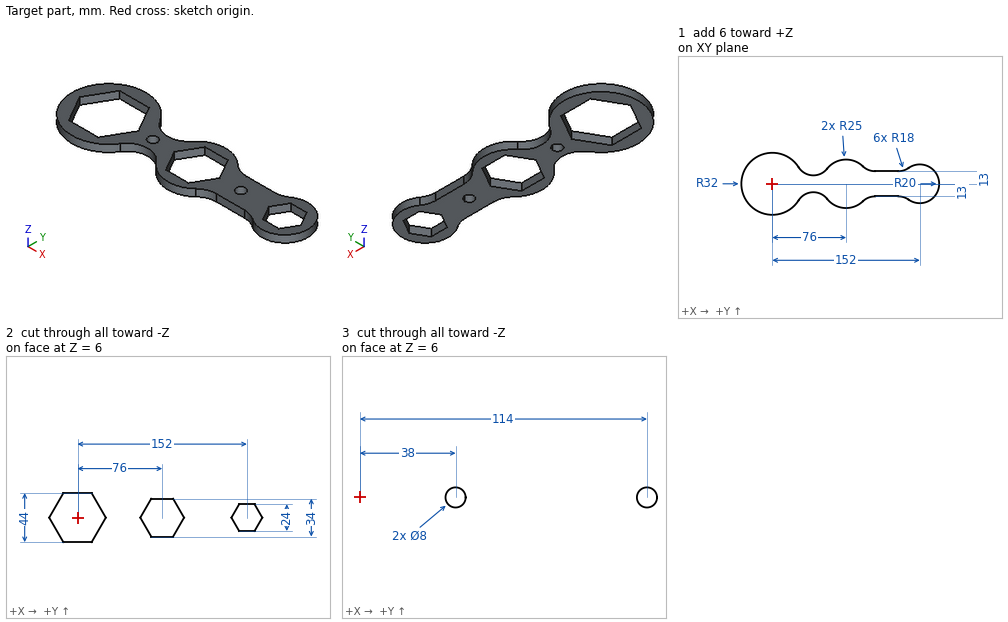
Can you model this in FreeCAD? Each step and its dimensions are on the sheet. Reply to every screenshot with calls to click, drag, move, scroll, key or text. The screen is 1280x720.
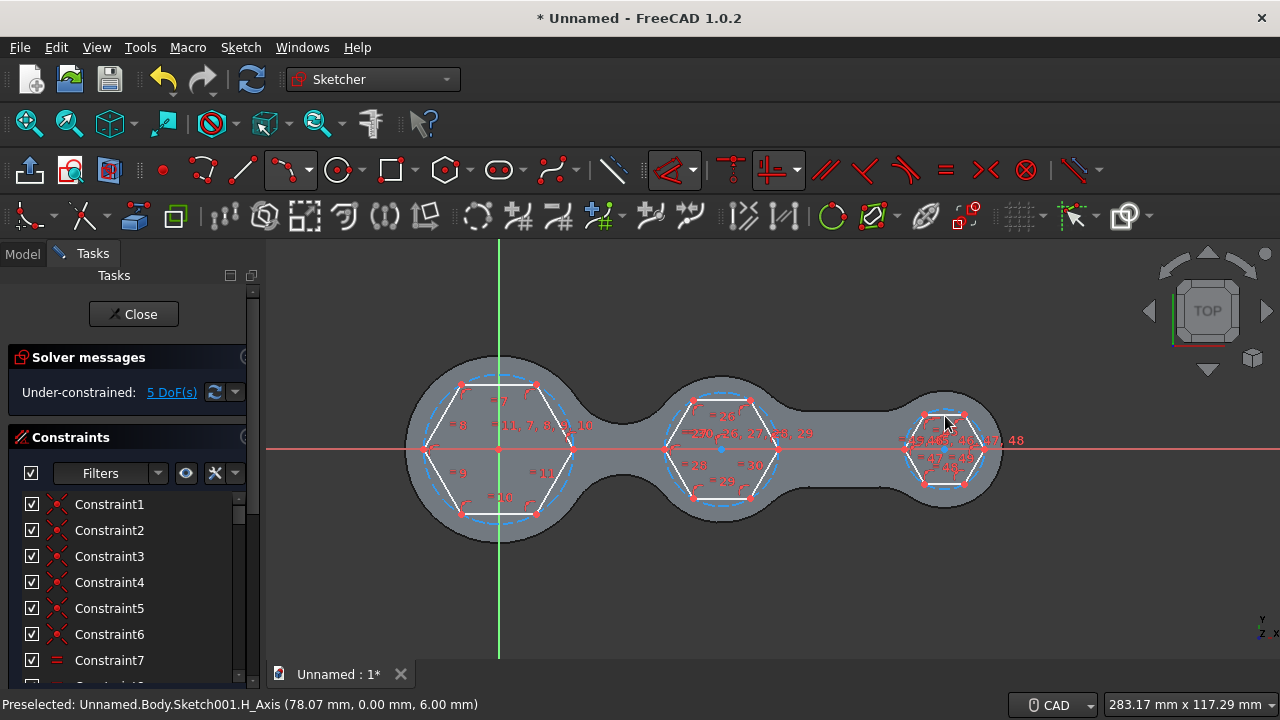
click(461, 514)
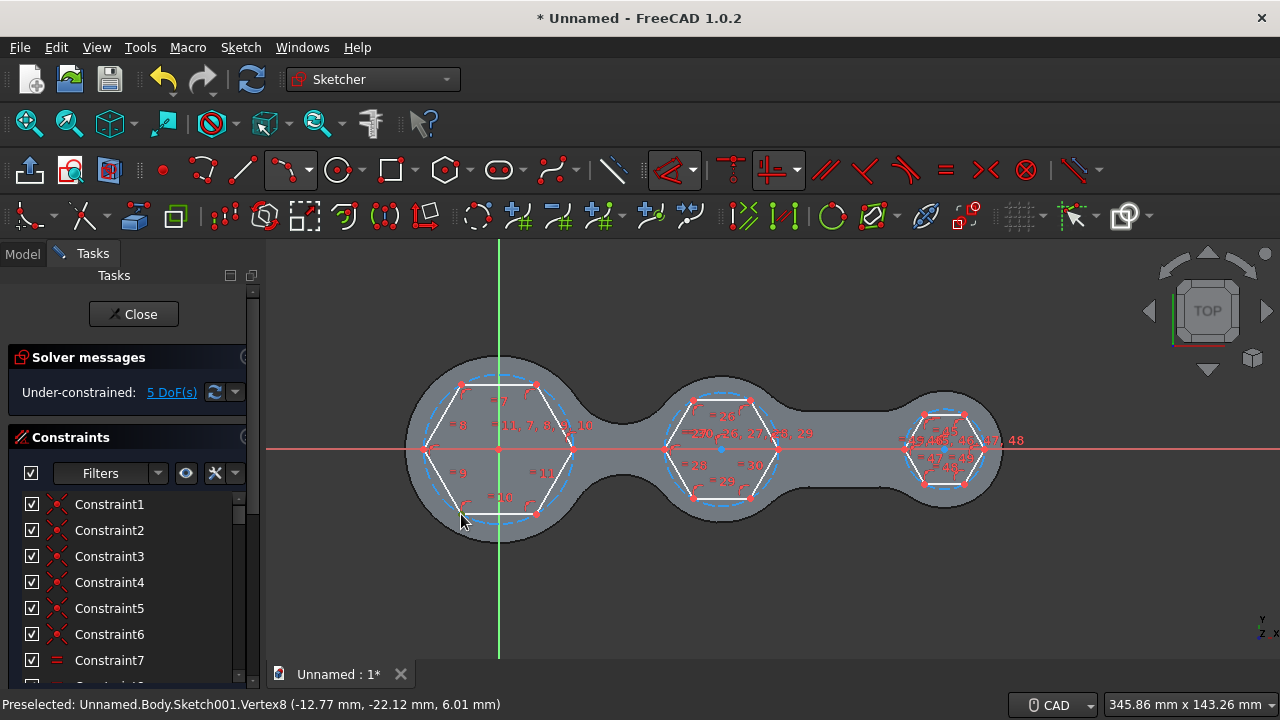
click(536, 385)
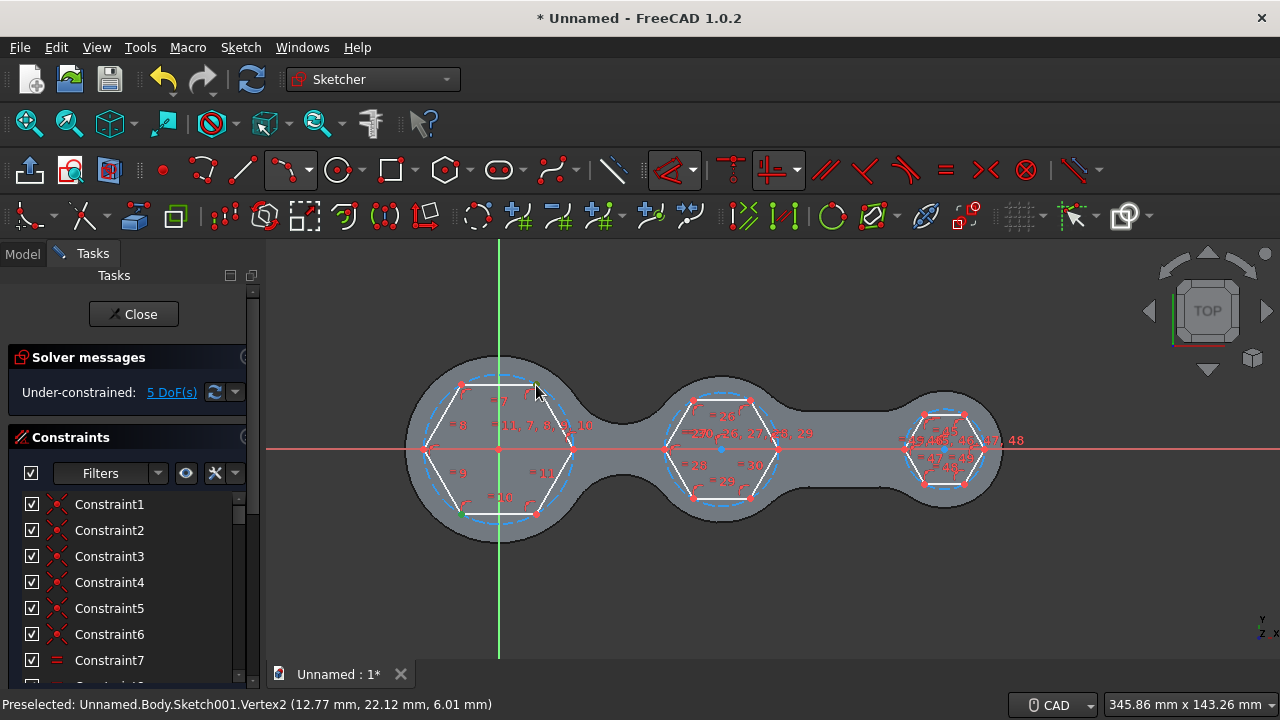
click(696, 170)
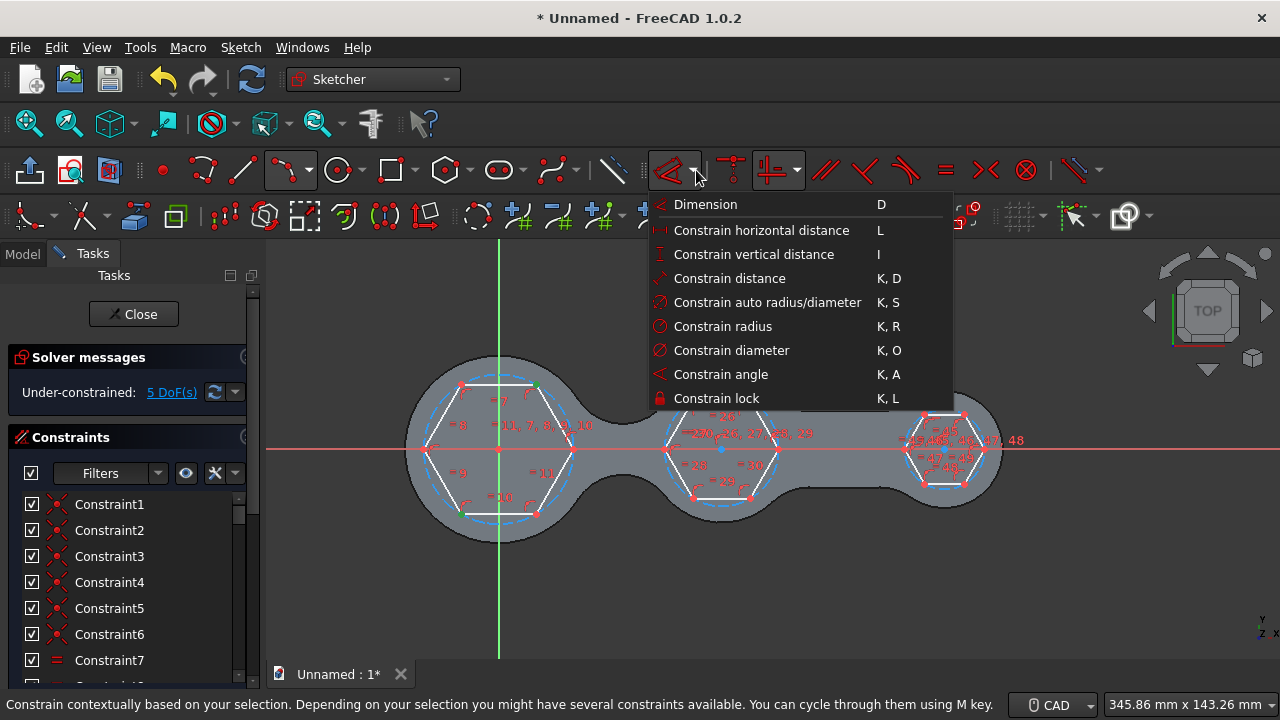
click(801, 254)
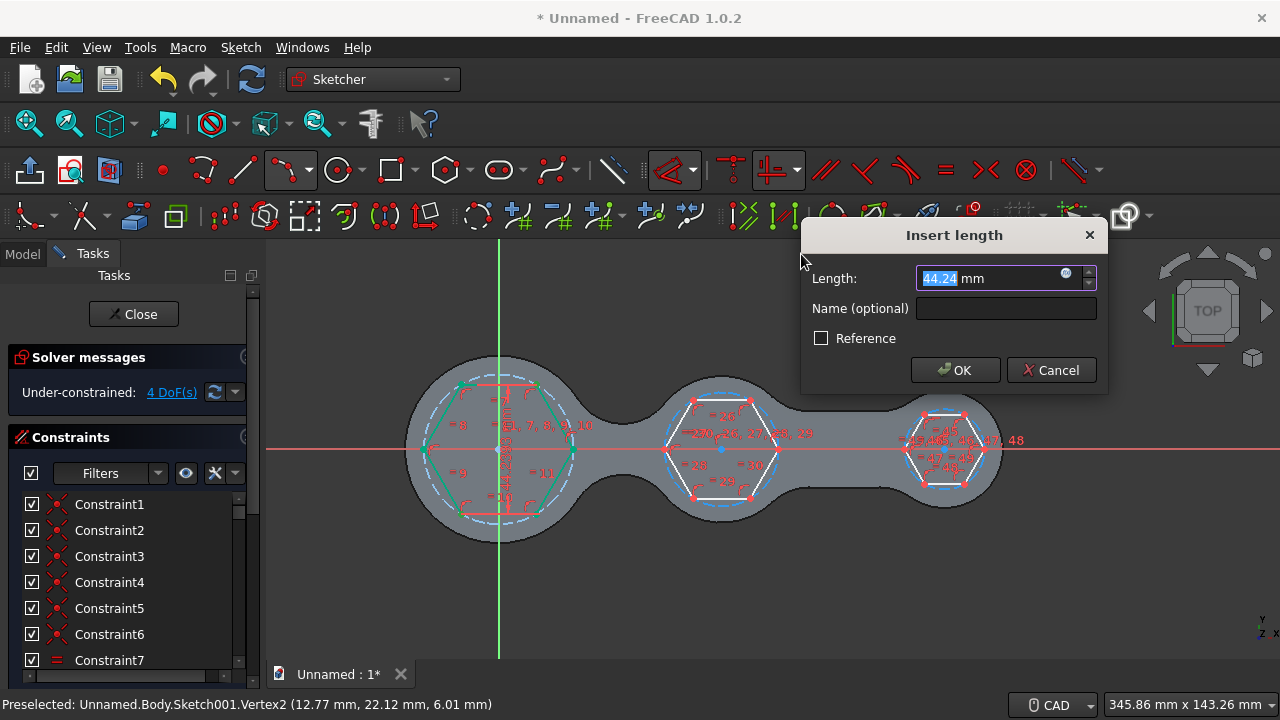
text(44)
key(Return)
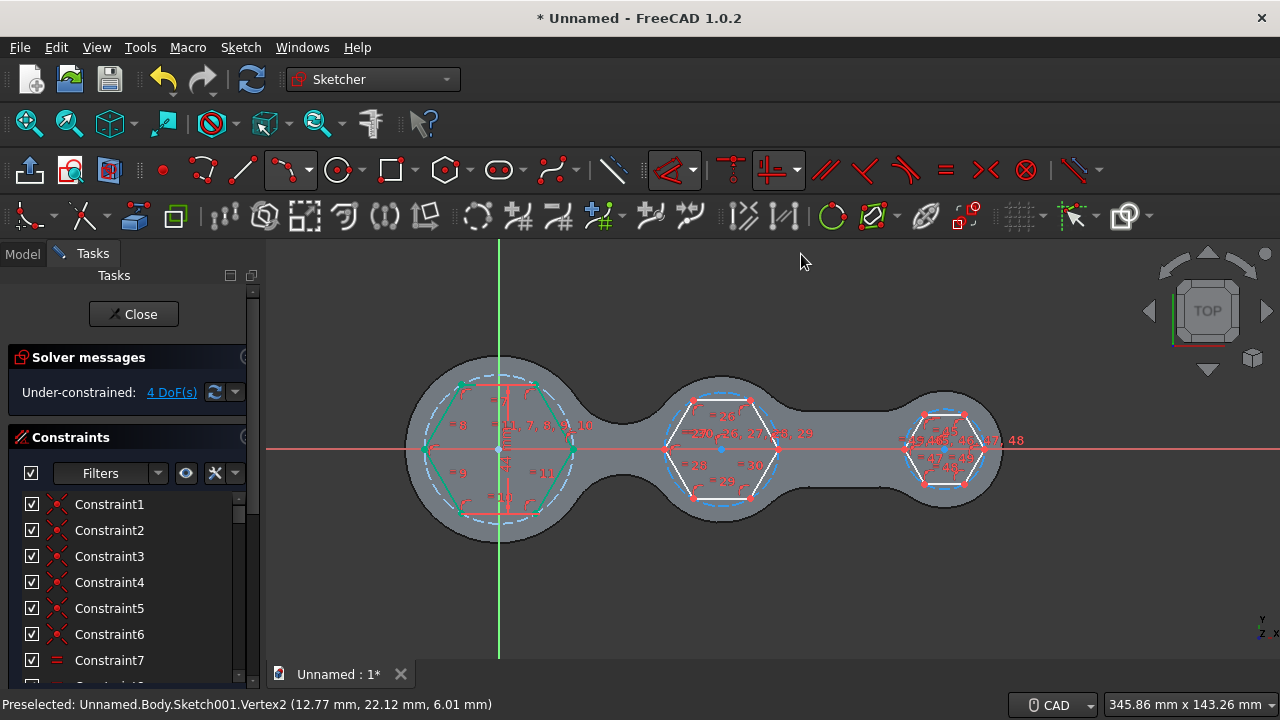
click(693, 499)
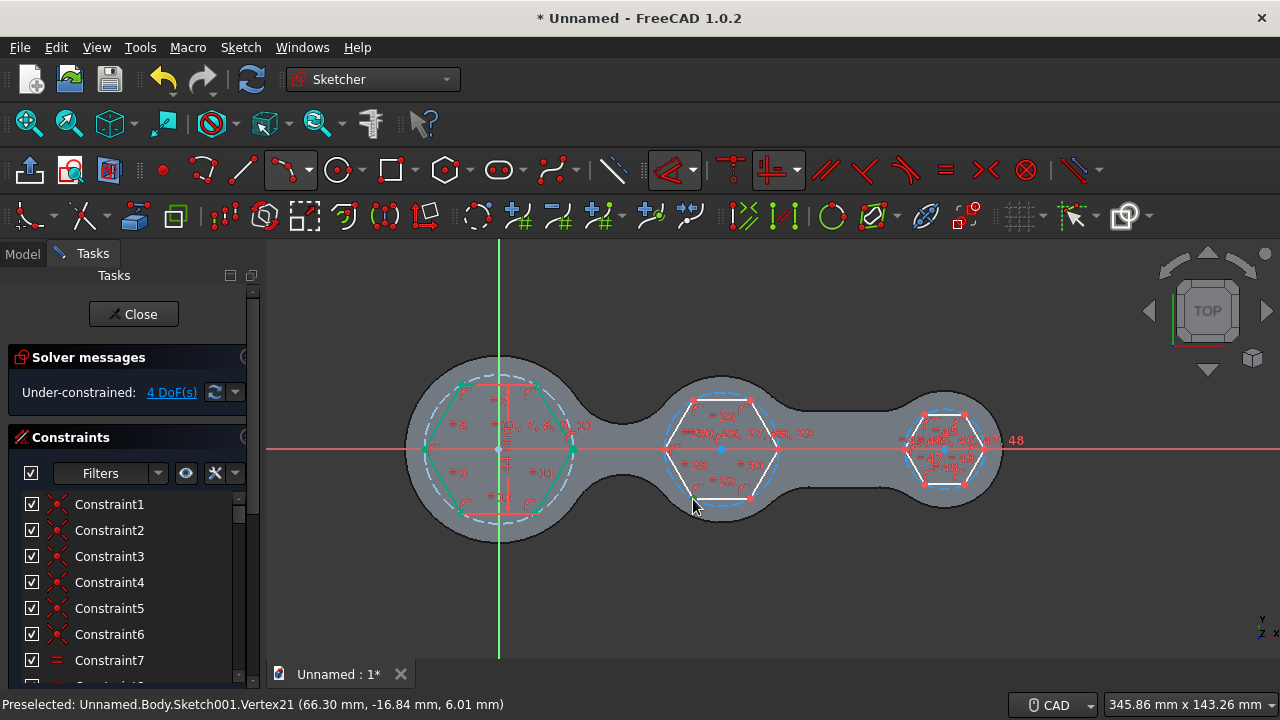
click(750, 400)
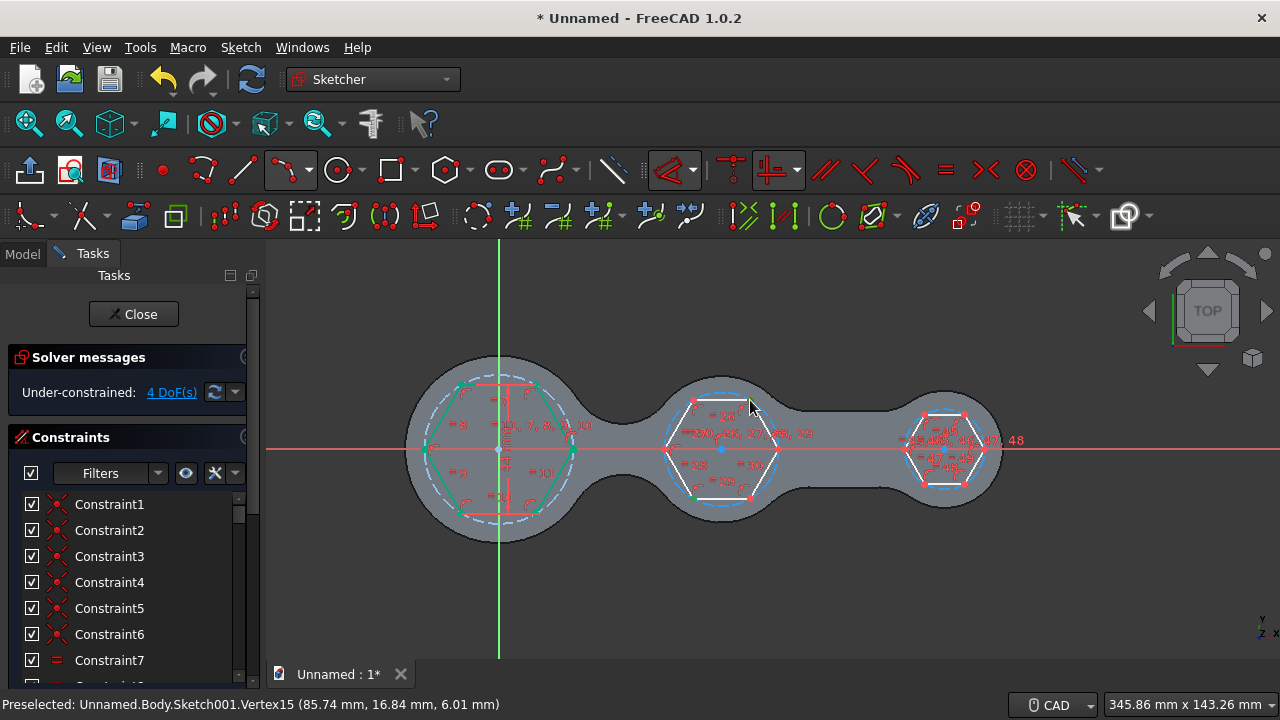
click(696, 170)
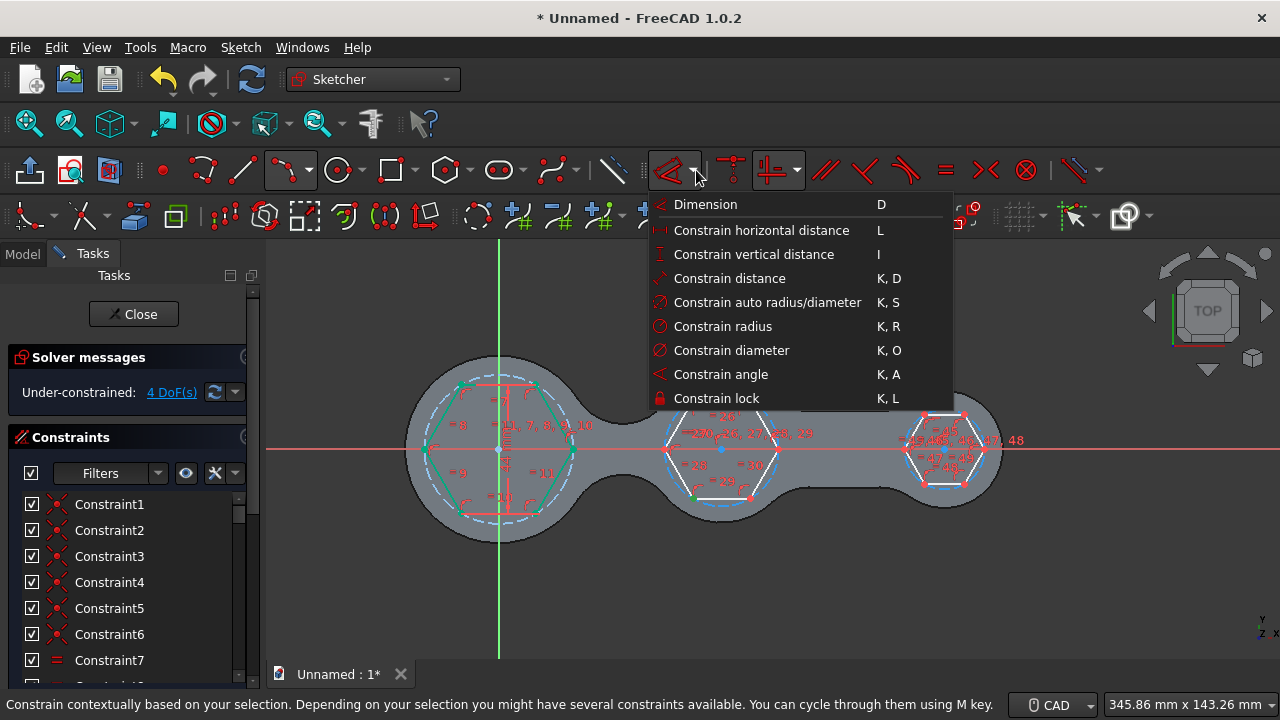
click(801, 254)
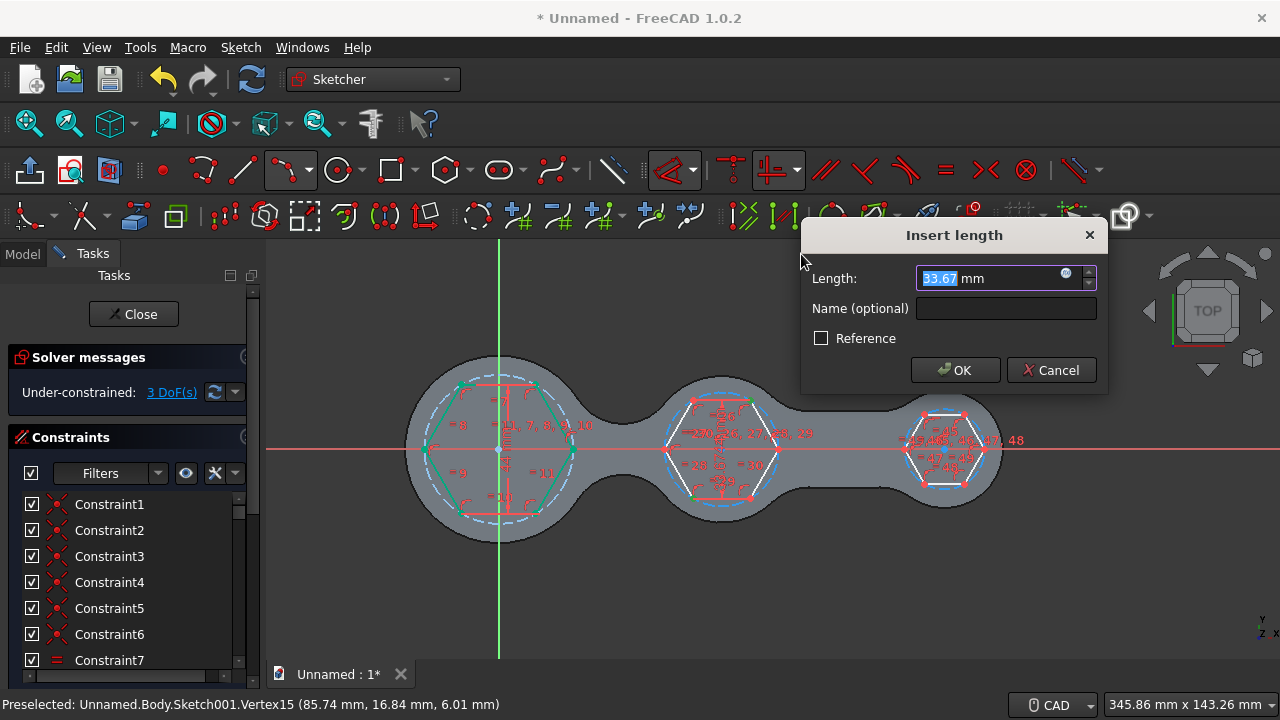
text(34)
key(Return)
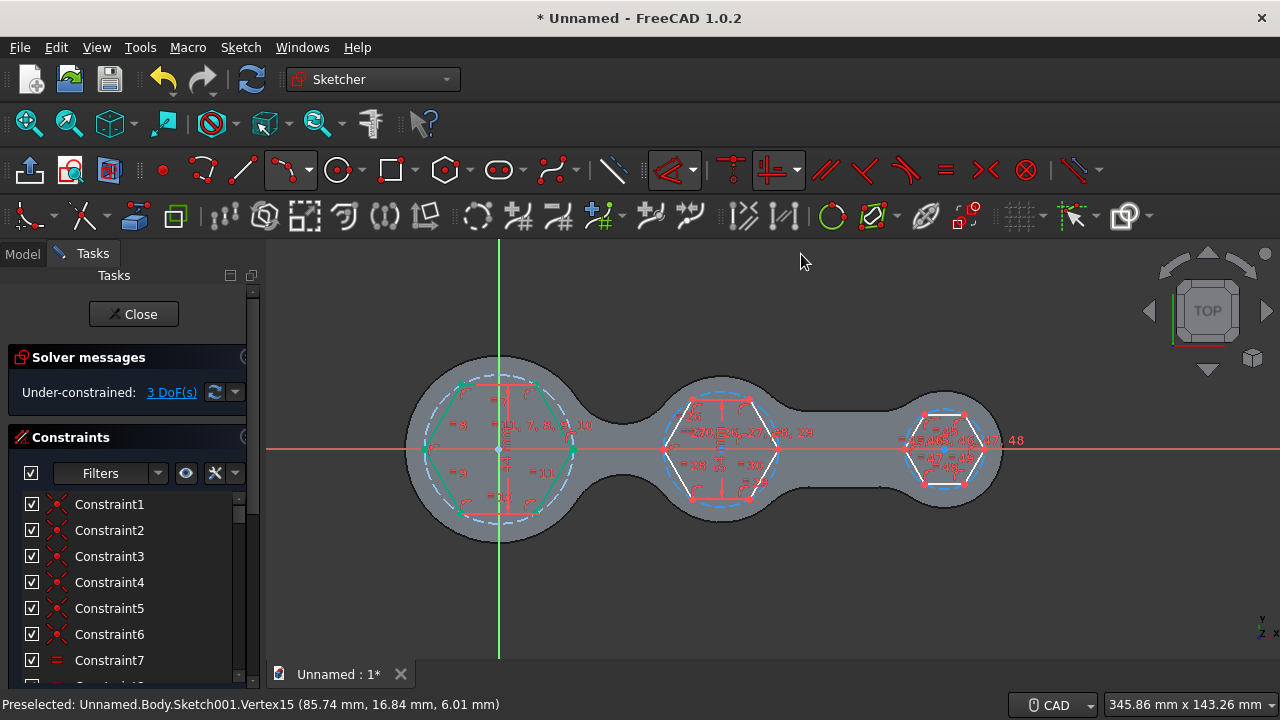
click(925, 484)